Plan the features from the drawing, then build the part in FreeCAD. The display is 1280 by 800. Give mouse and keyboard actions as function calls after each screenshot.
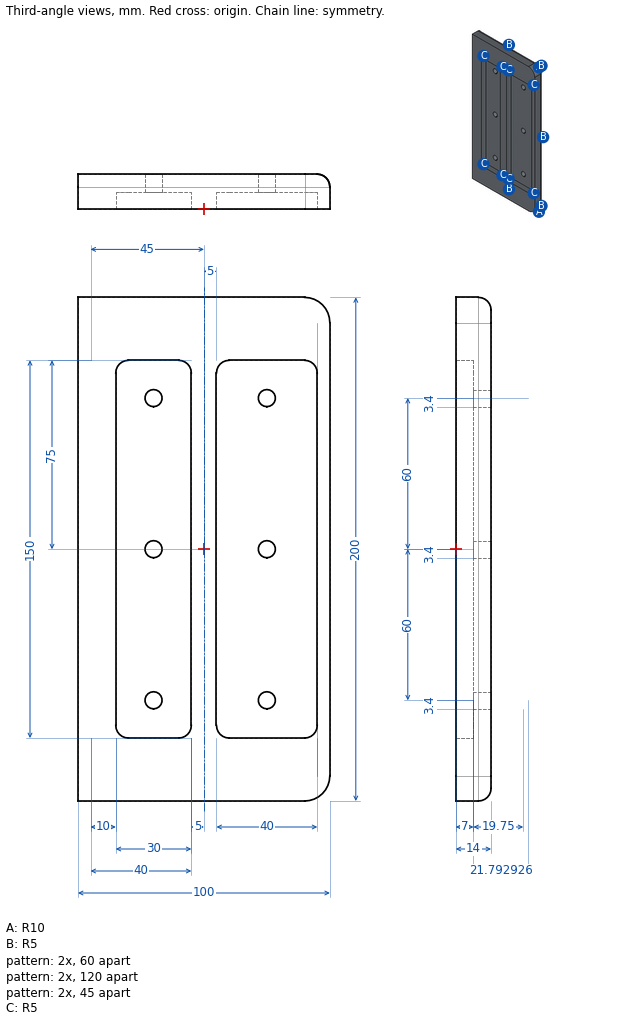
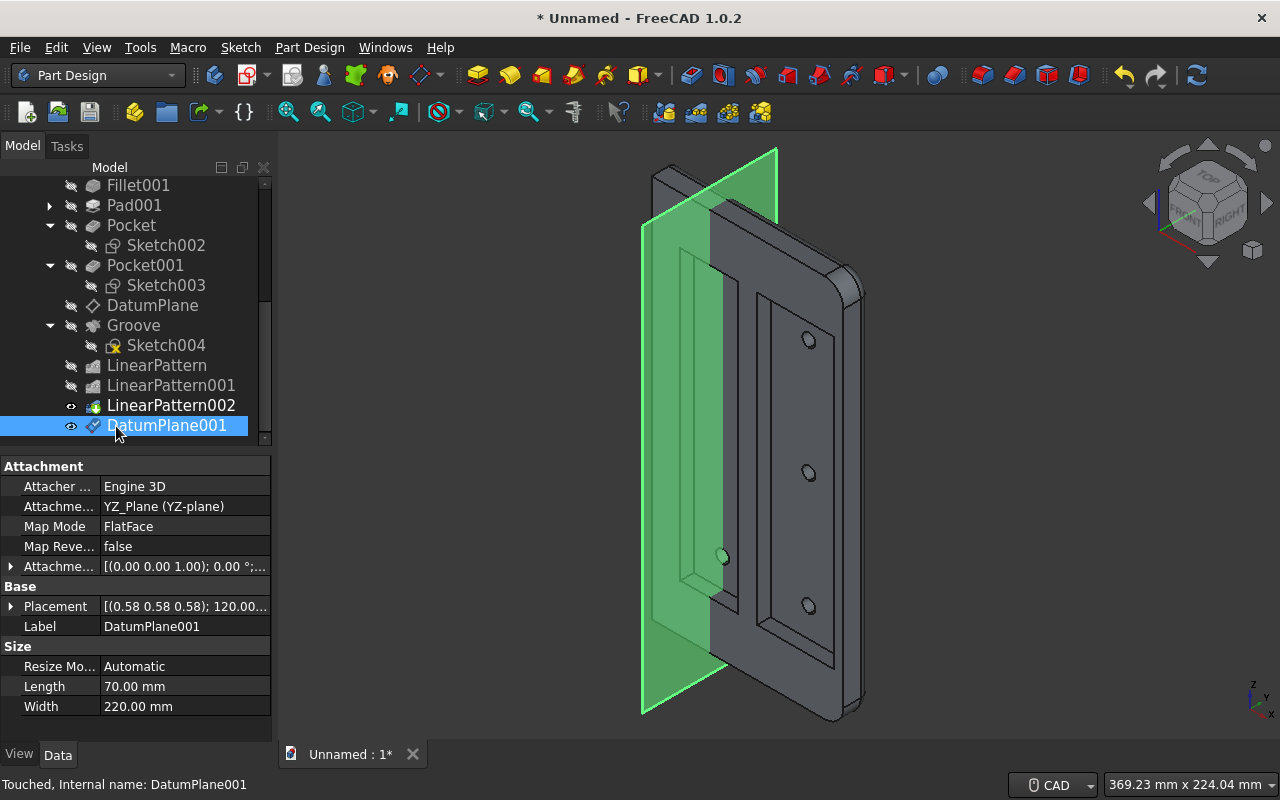
click(248, 76)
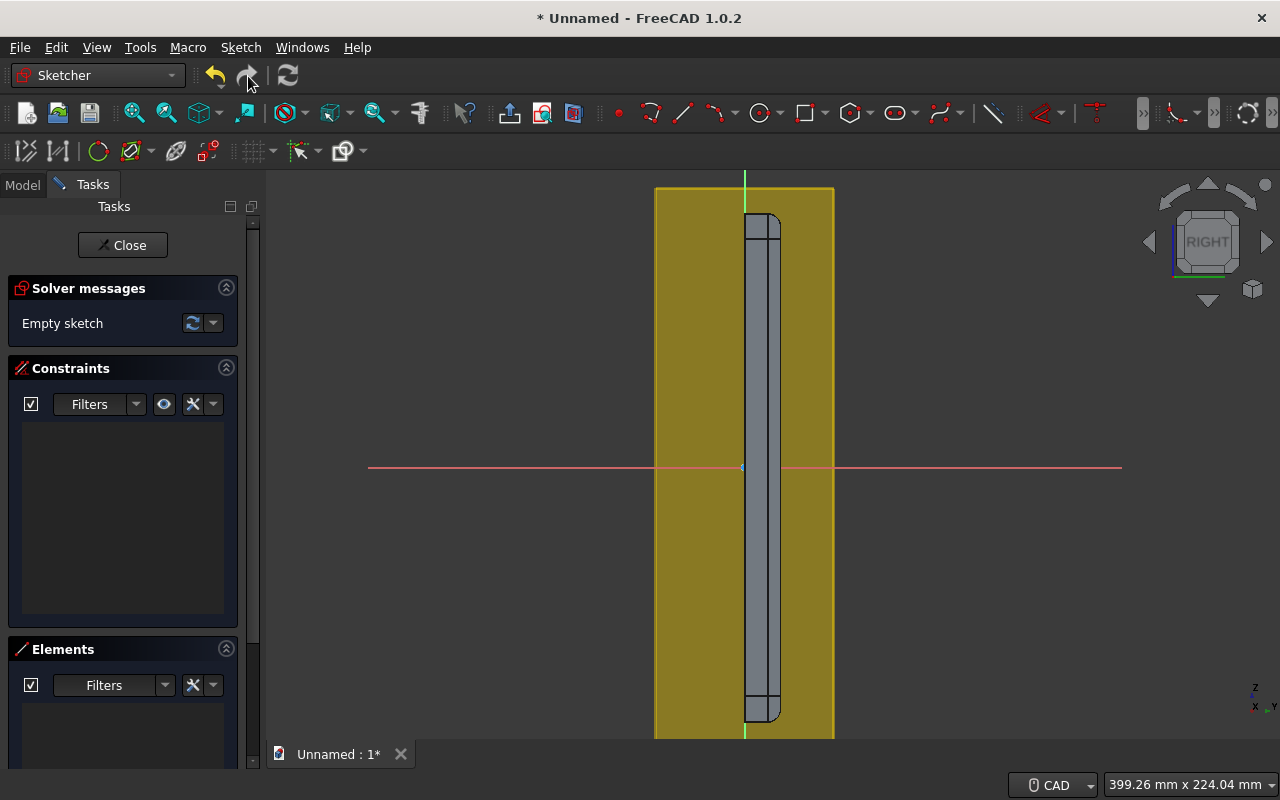
click(574, 114)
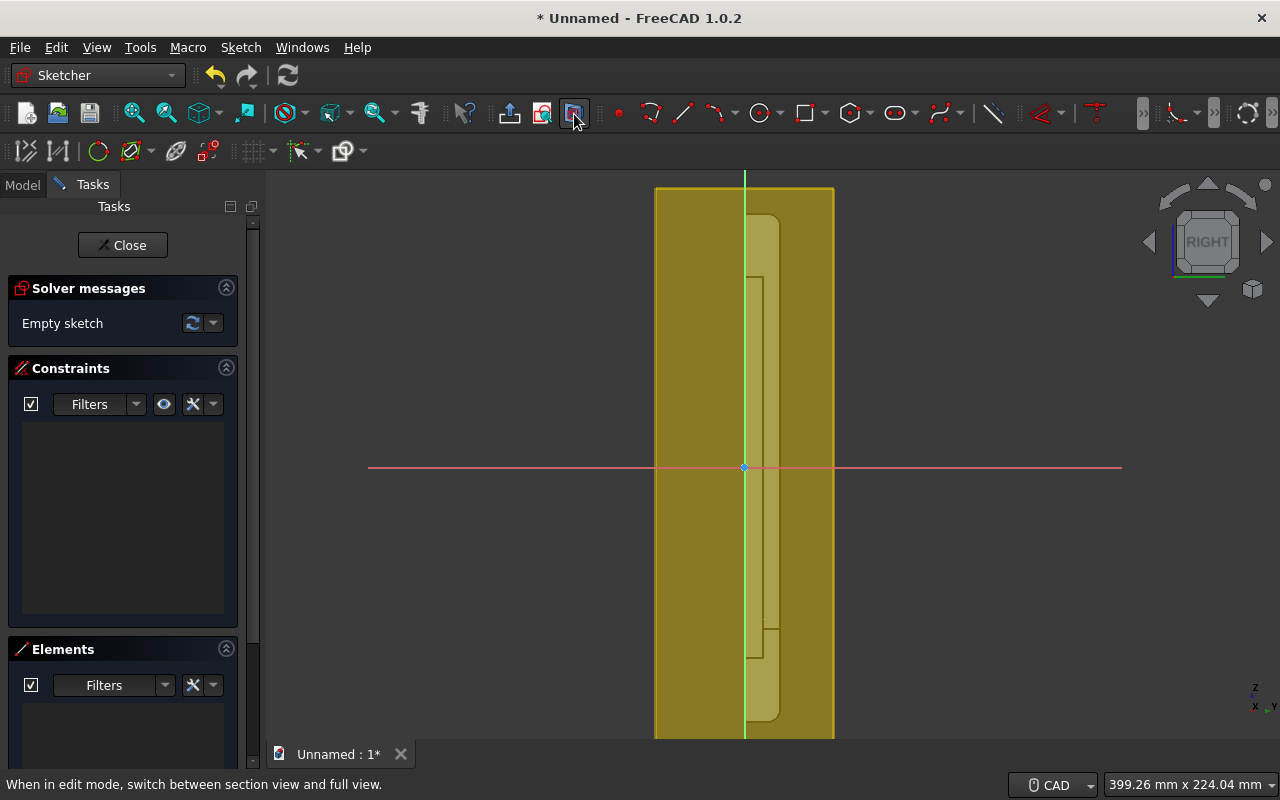
scroll(793, 475, up, 10)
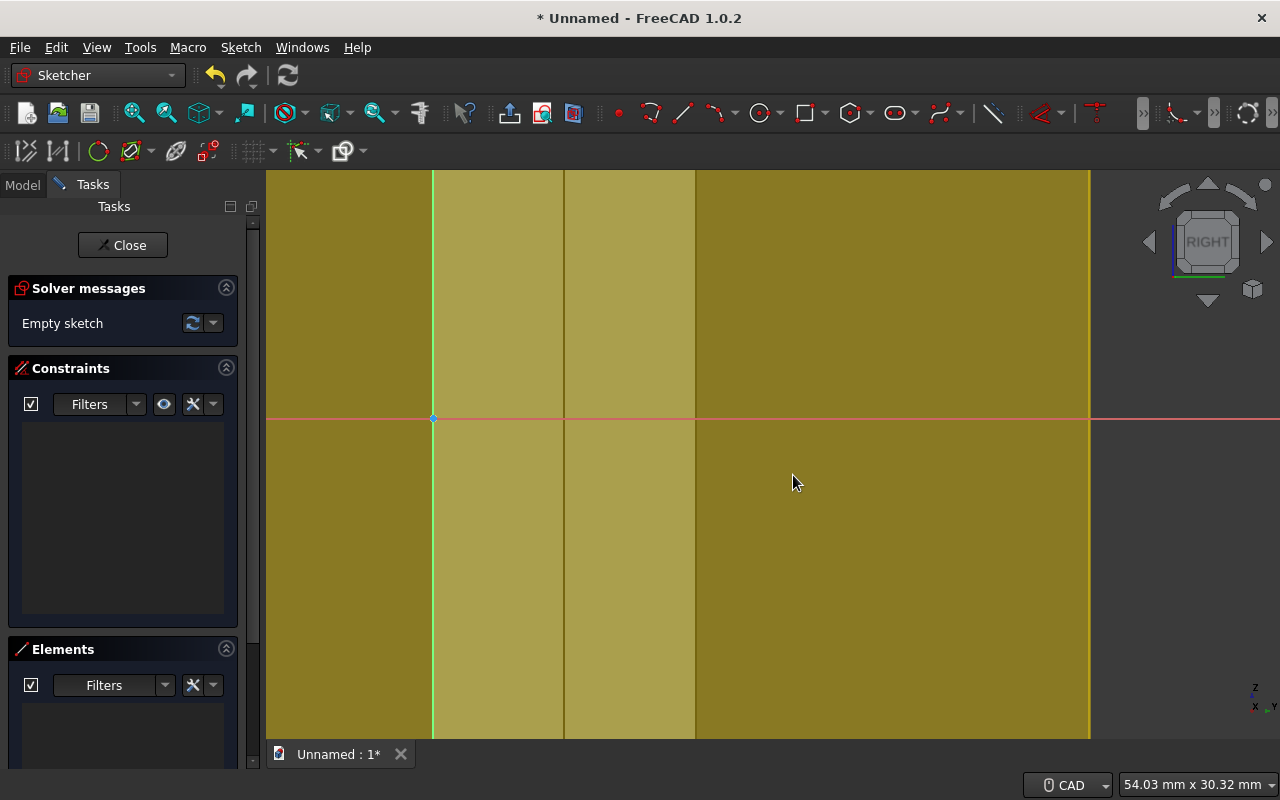
click(652, 114)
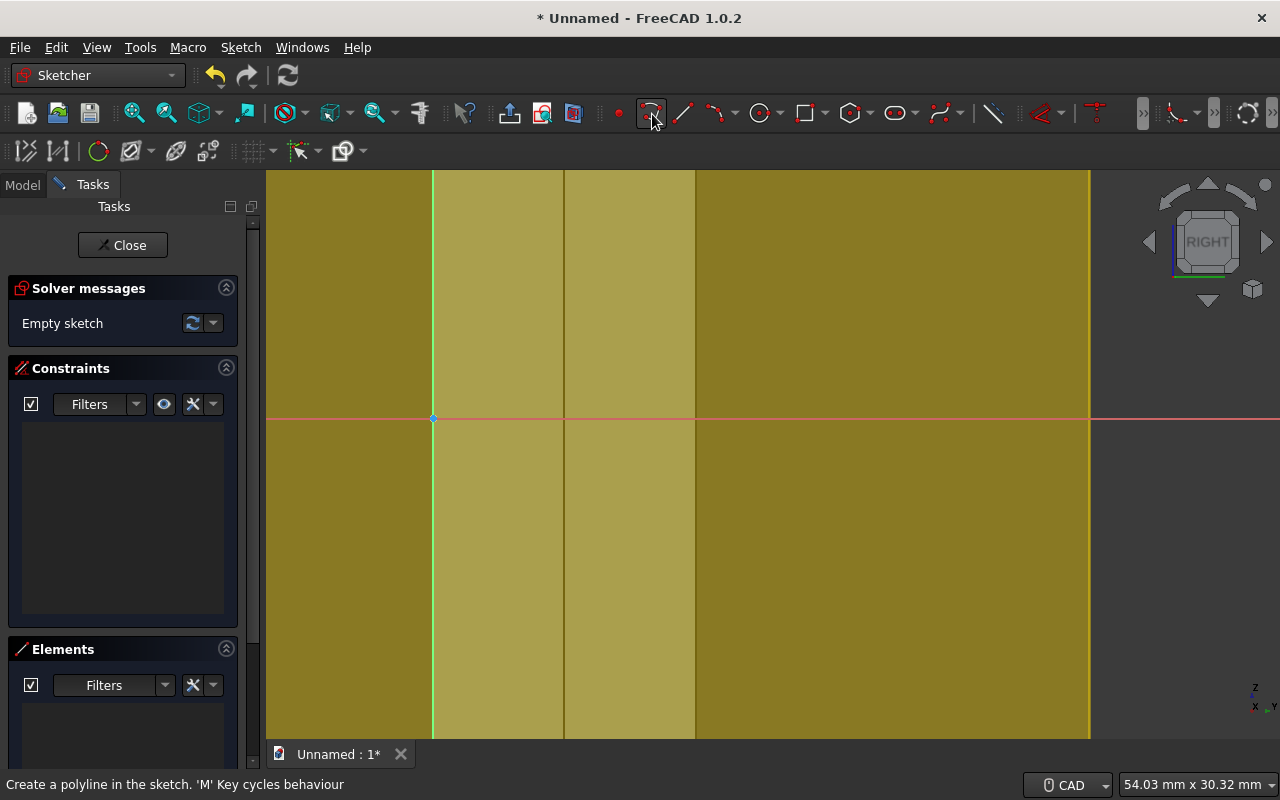
click(564, 419)
click(564, 483)
click(935, 483)
click(973, 428)
click(564, 419)
key(Escape)
key(Escape)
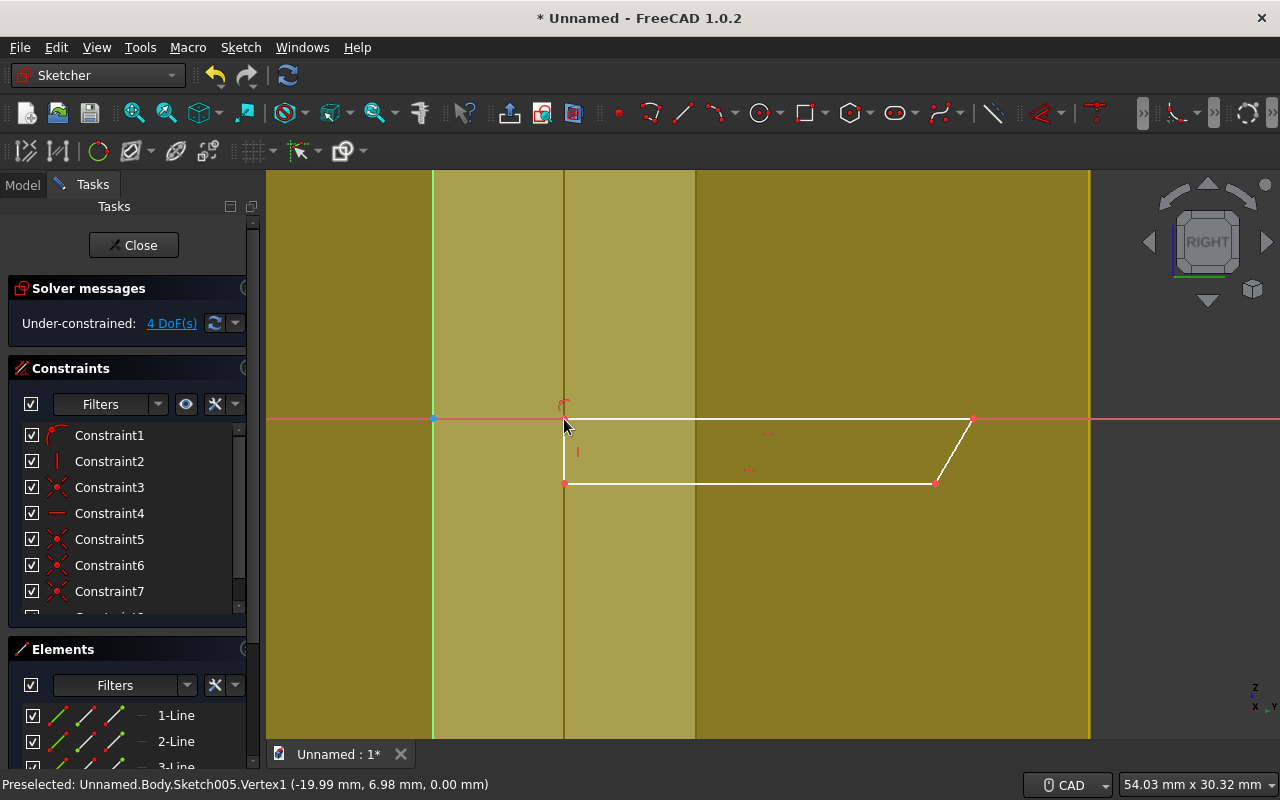
key(d)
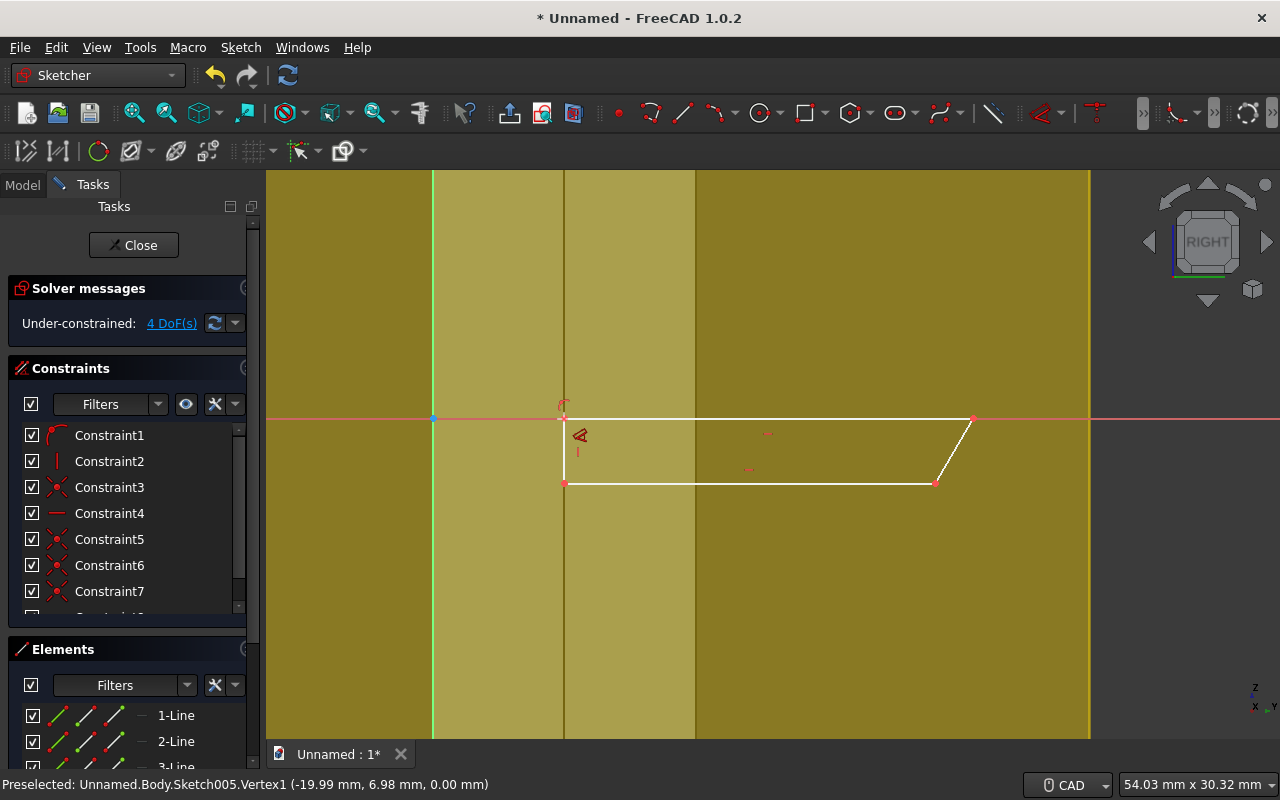
click(564, 419)
click(499, 385)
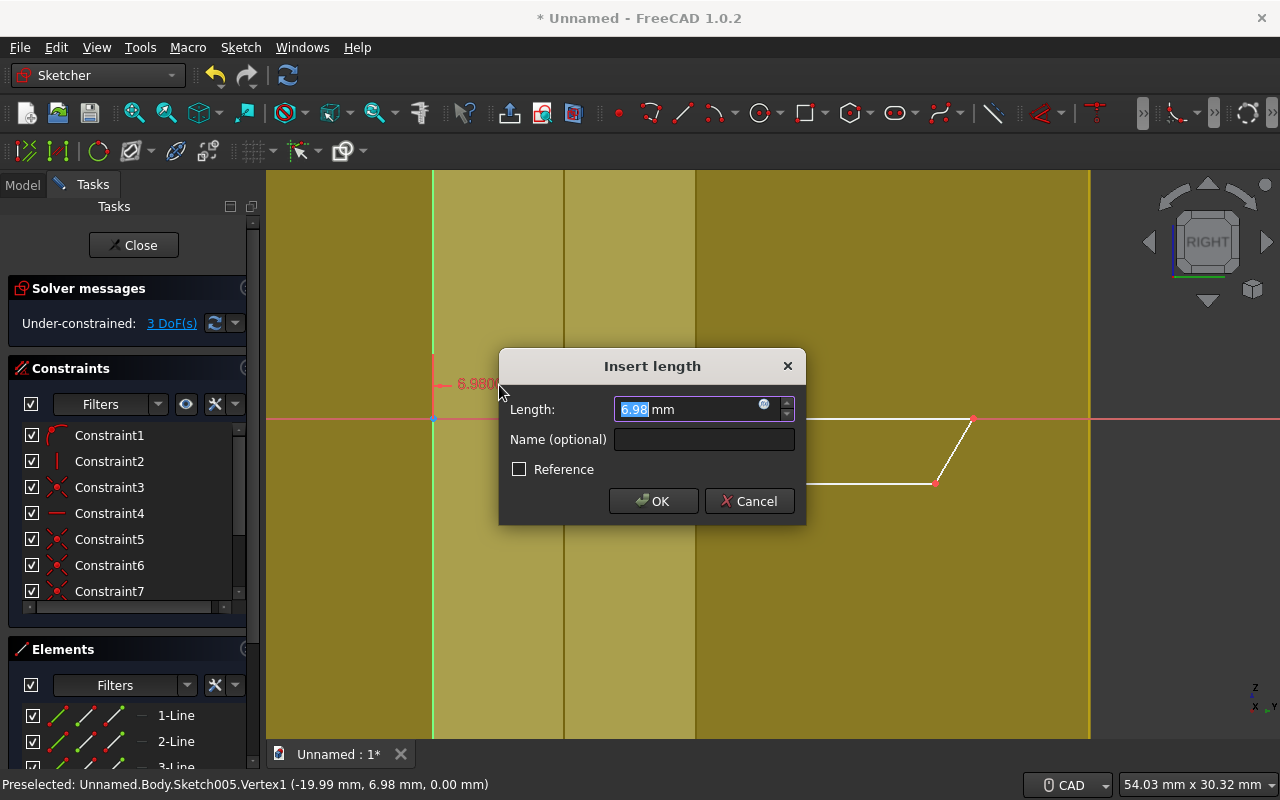
text(7)
key(Return)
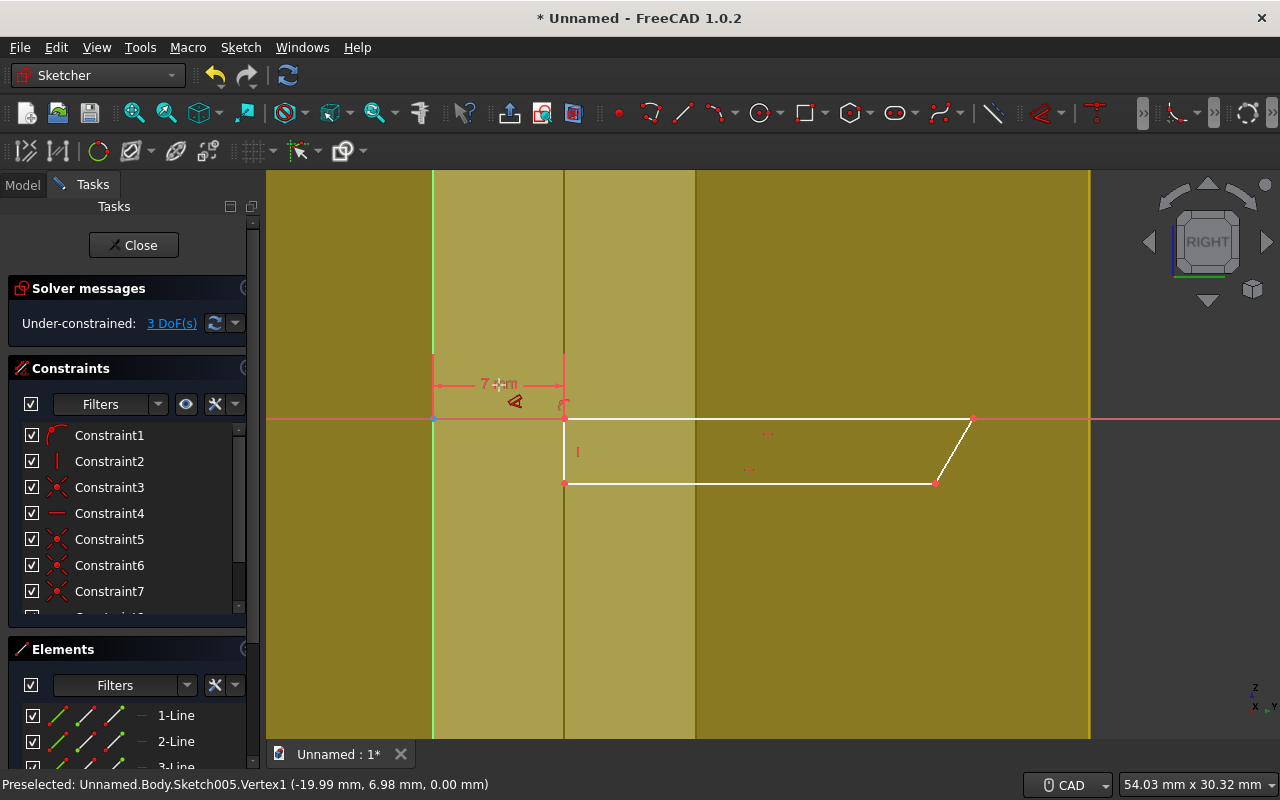
click(564, 438)
click(530, 451)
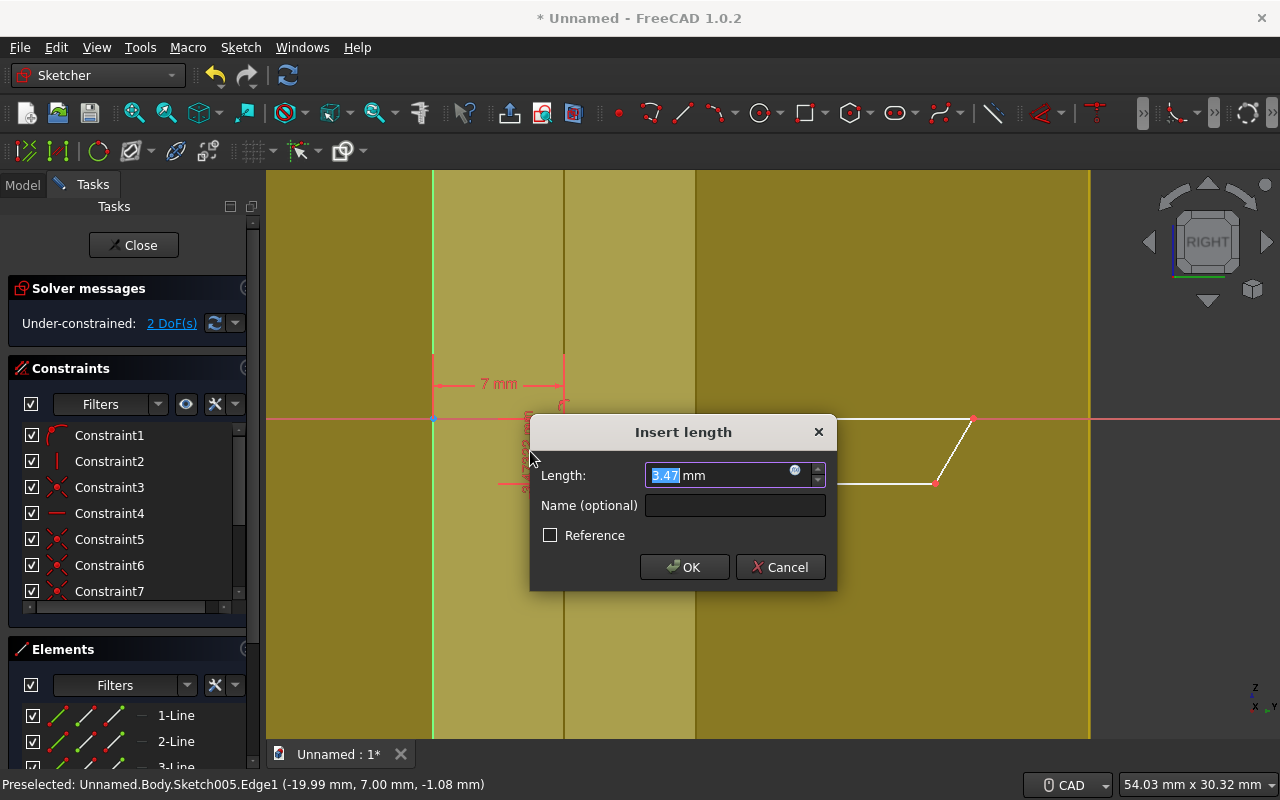
text(3.4)
key(Return)